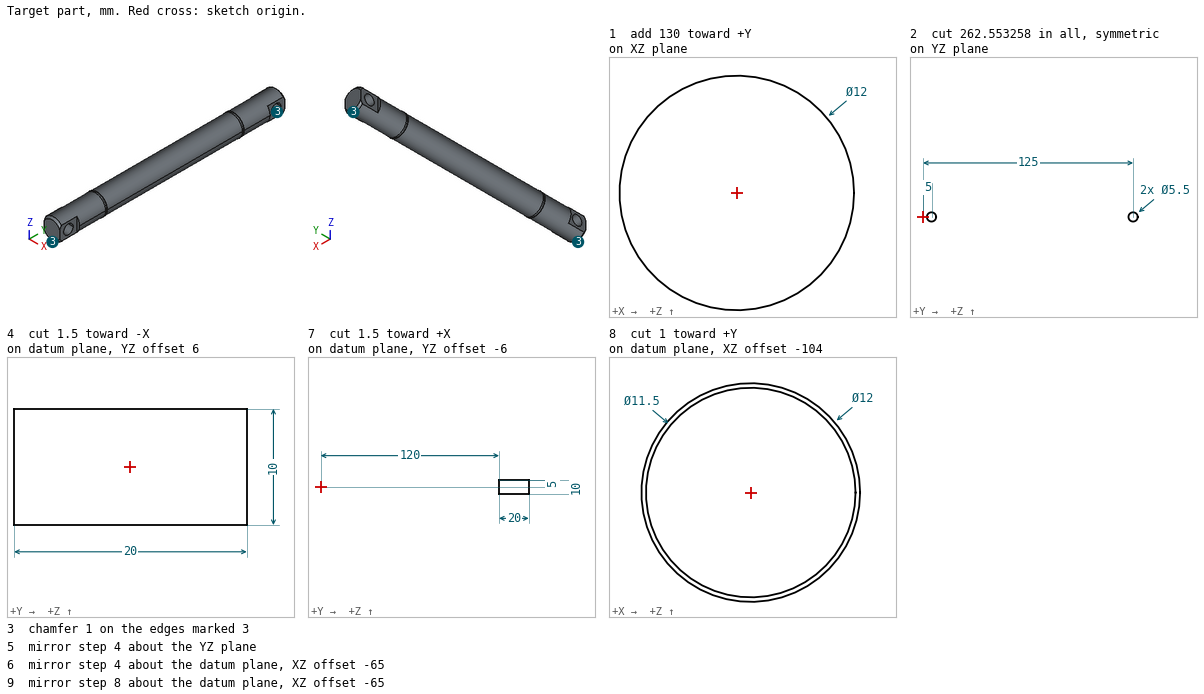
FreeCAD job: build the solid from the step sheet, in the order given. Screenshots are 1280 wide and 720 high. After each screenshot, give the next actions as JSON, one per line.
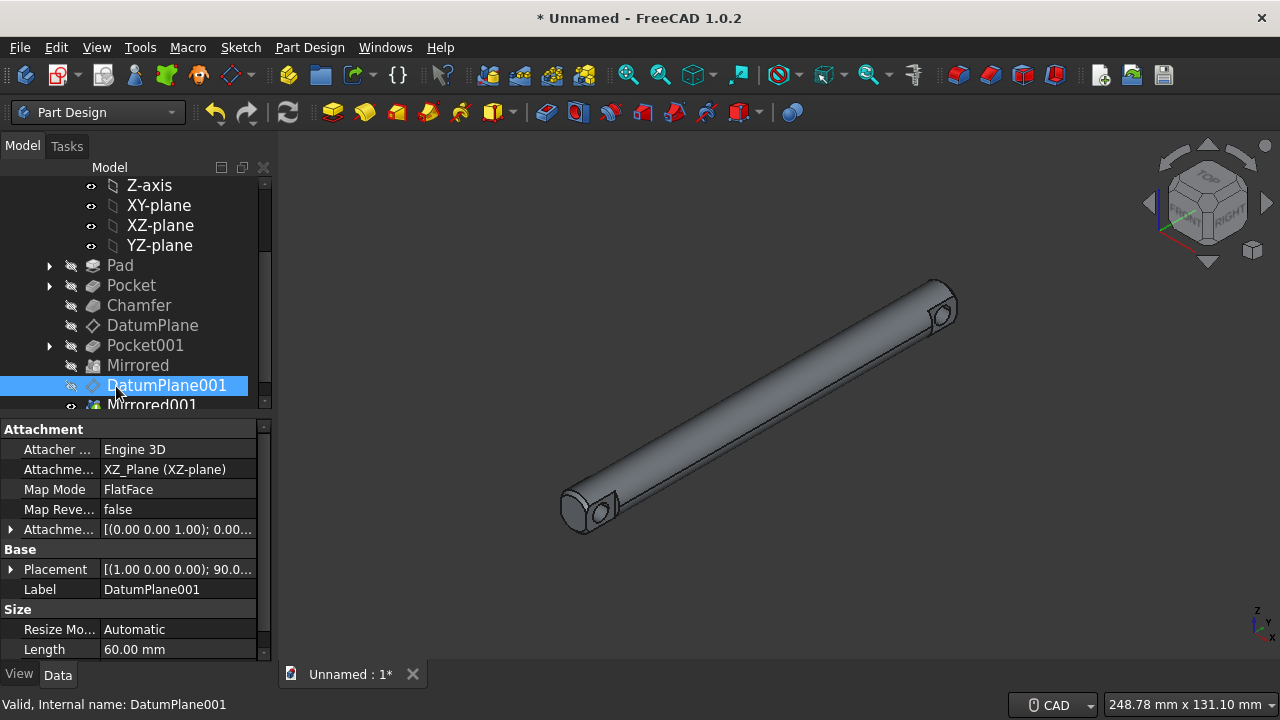
{"action": "scroll", "coordinate": [160, 301], "scroll_direction": "down", "scroll_amount": 3}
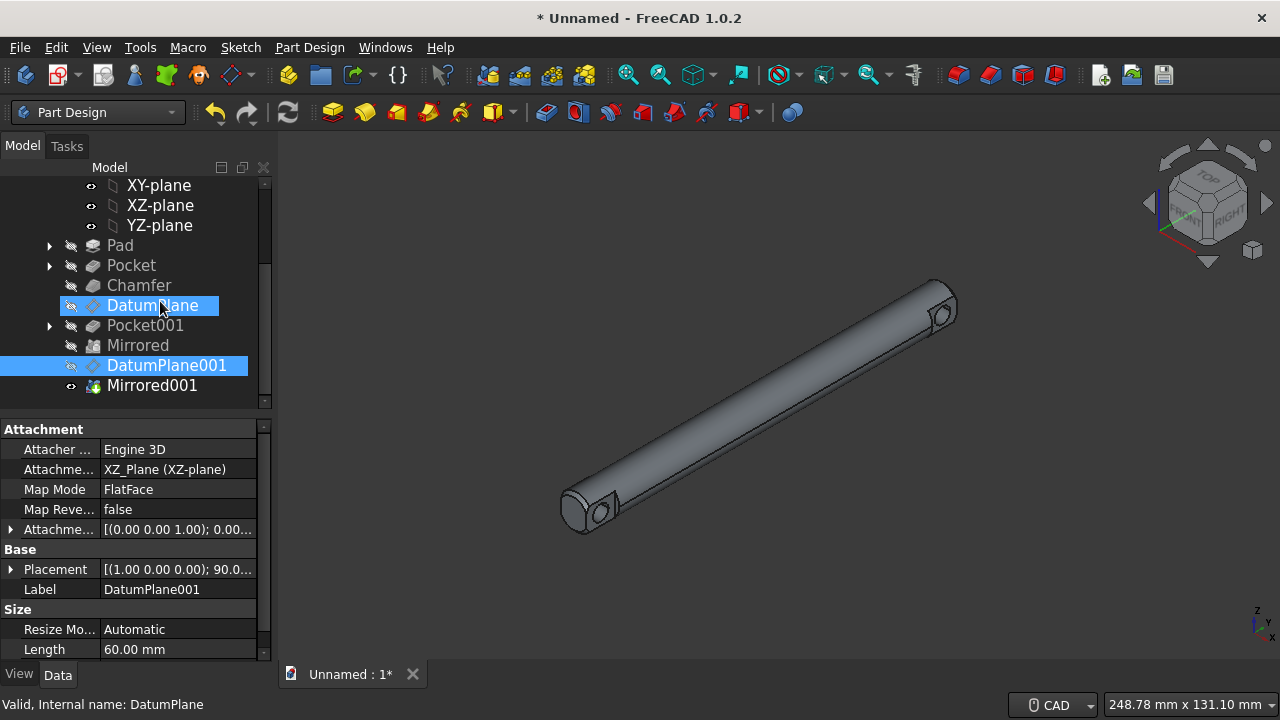
{"action": "scroll", "coordinate": [160, 281], "scroll_direction": "up", "scroll_amount": 15}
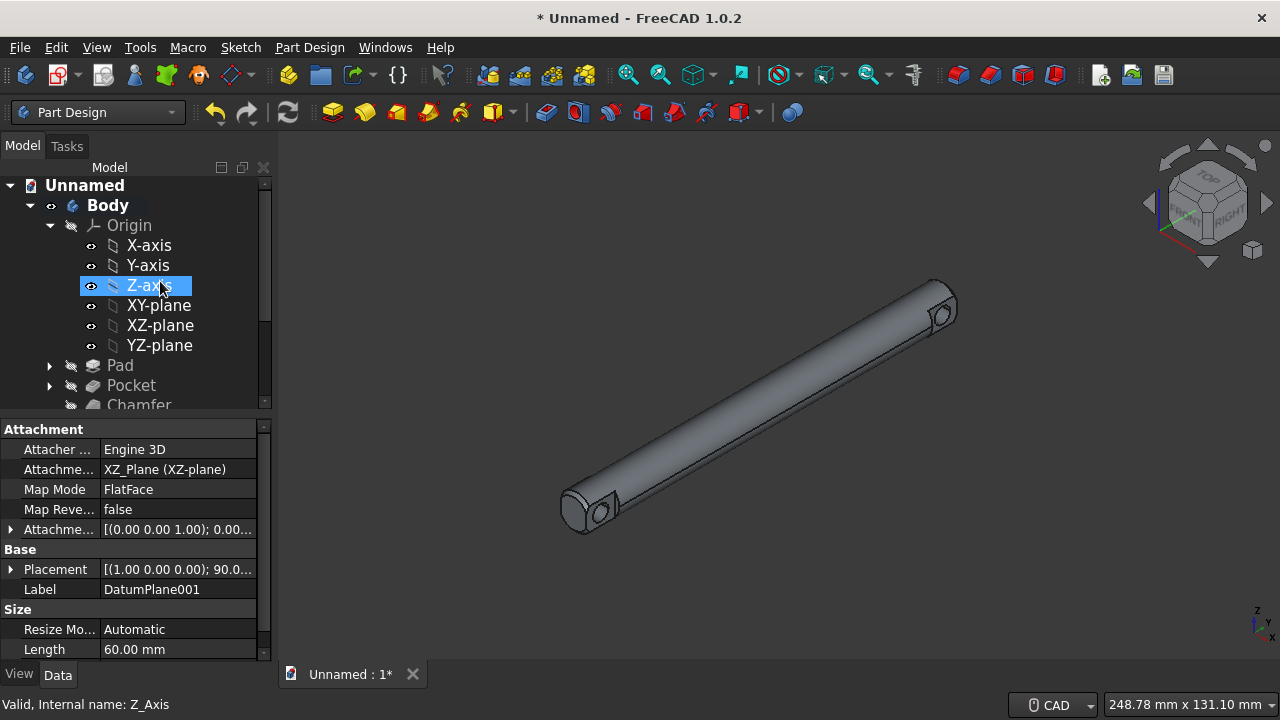
{"action": "left_click", "coordinate": [136, 346]}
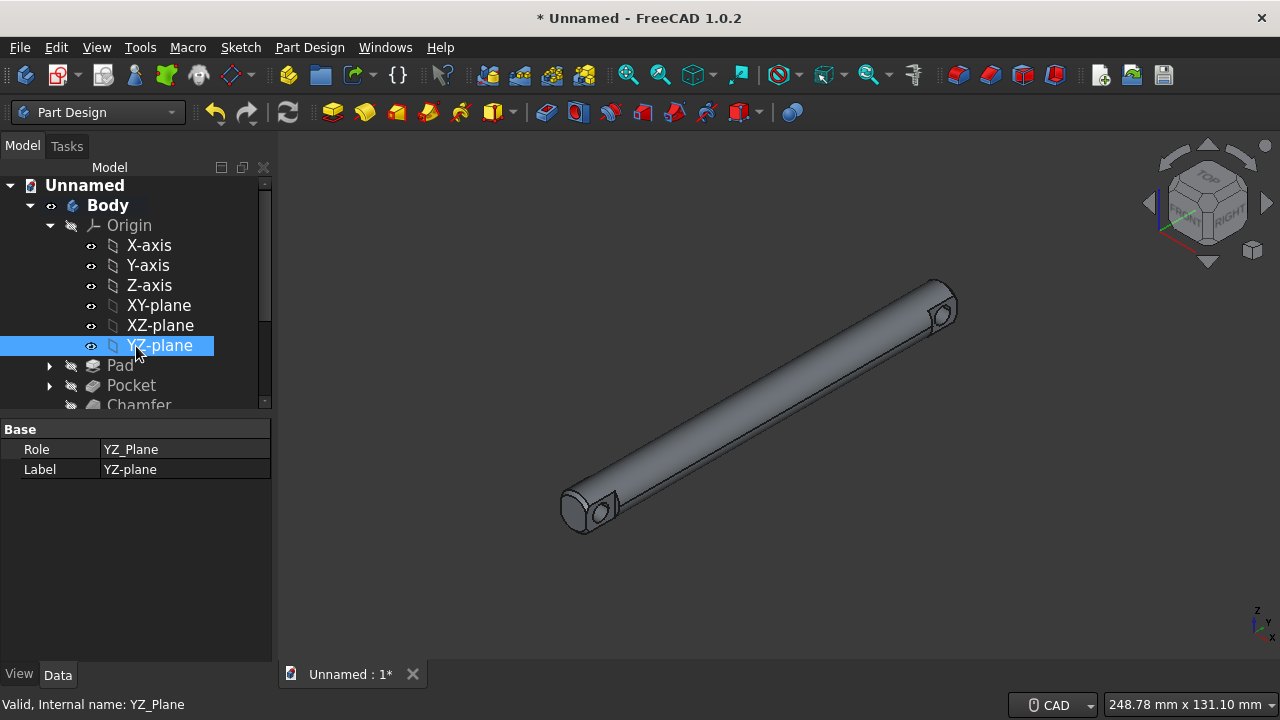
{"action": "left_click", "coordinate": [232, 76]}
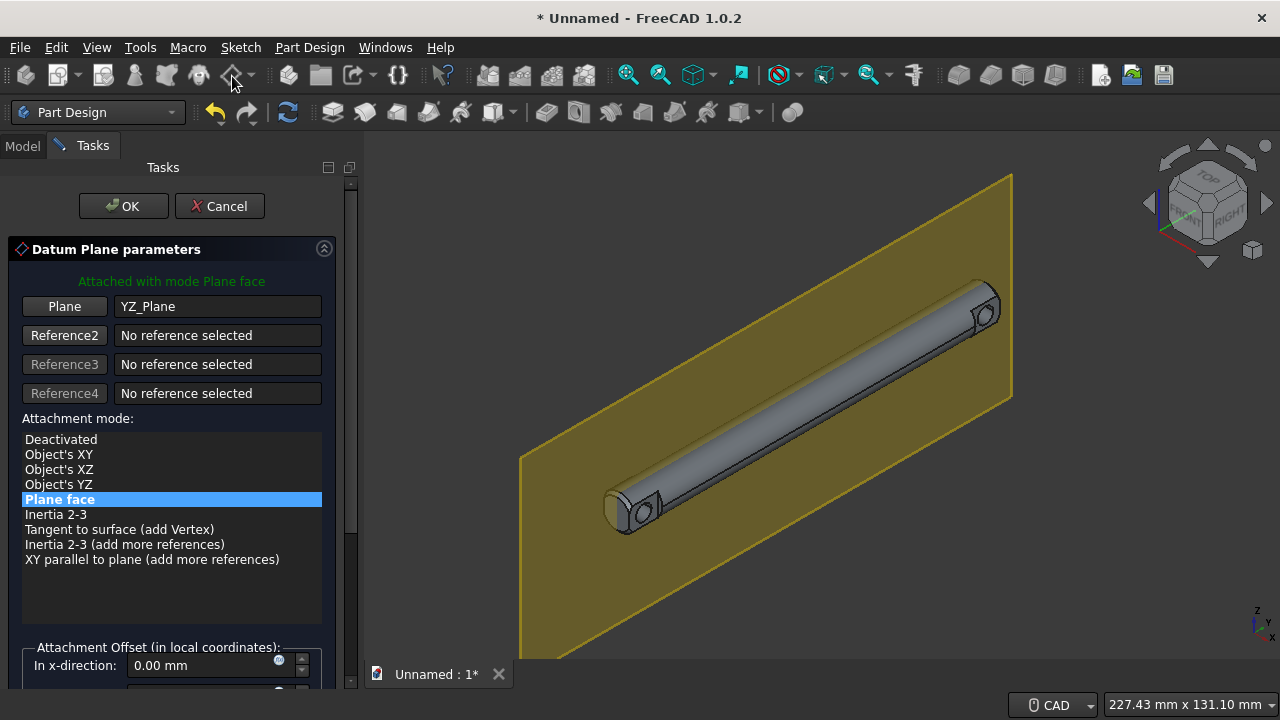
{"action": "scroll", "coordinate": [351, 432], "scroll_direction": "down", "scroll_amount": 2}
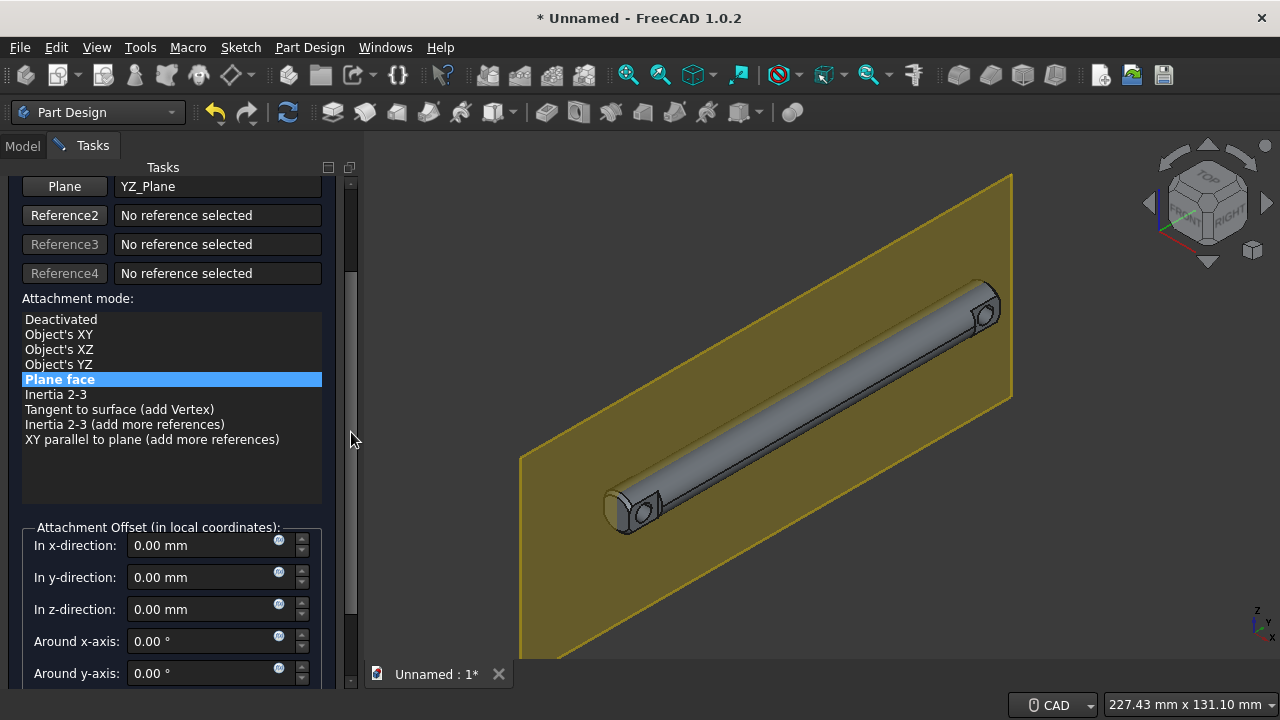
{"action": "triple_click", "coordinate": [210, 609]}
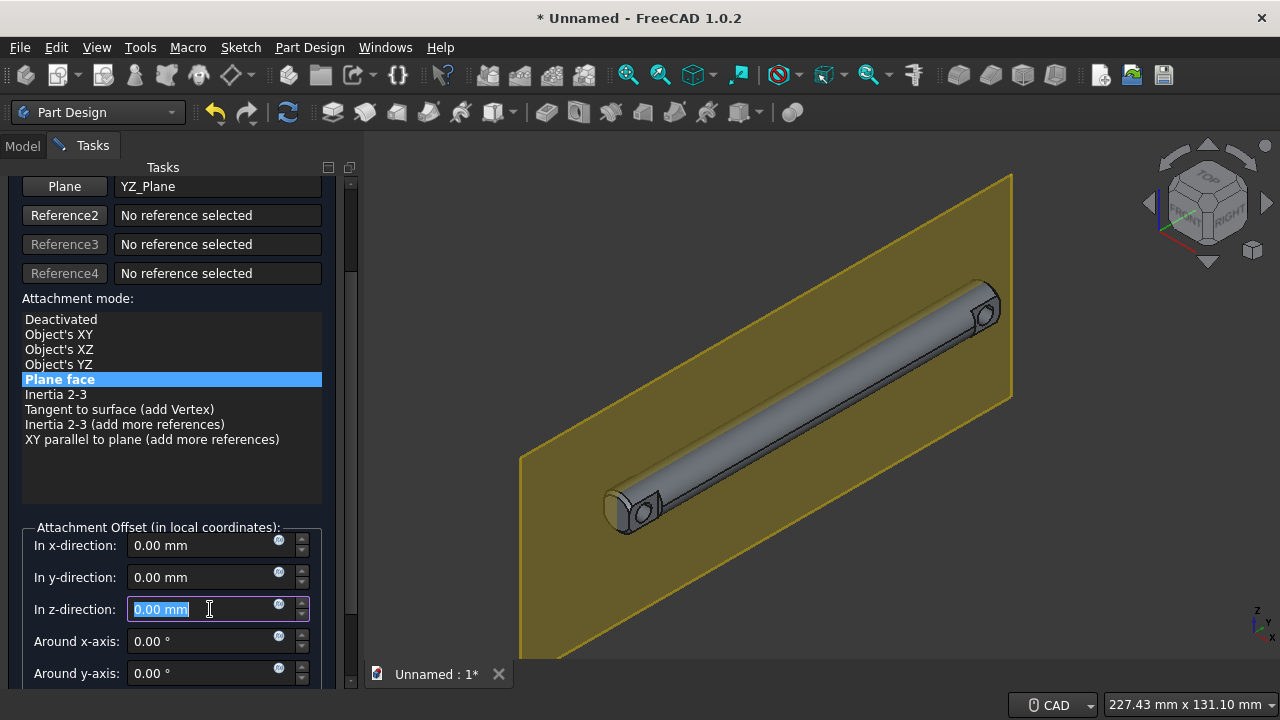
{"action": "type", "text": "-6"}
{"action": "key", "text": "Tab"}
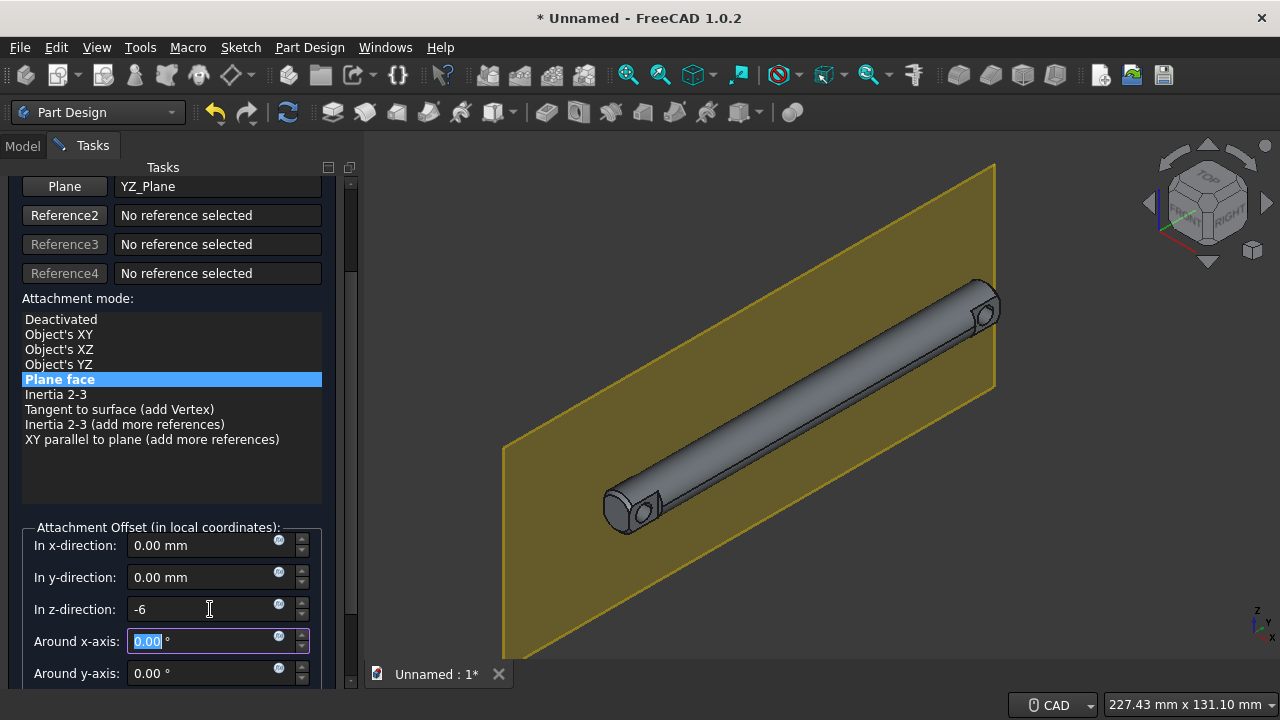
{"action": "scroll", "coordinate": [351, 432], "scroll_direction": "up", "scroll_amount": 3}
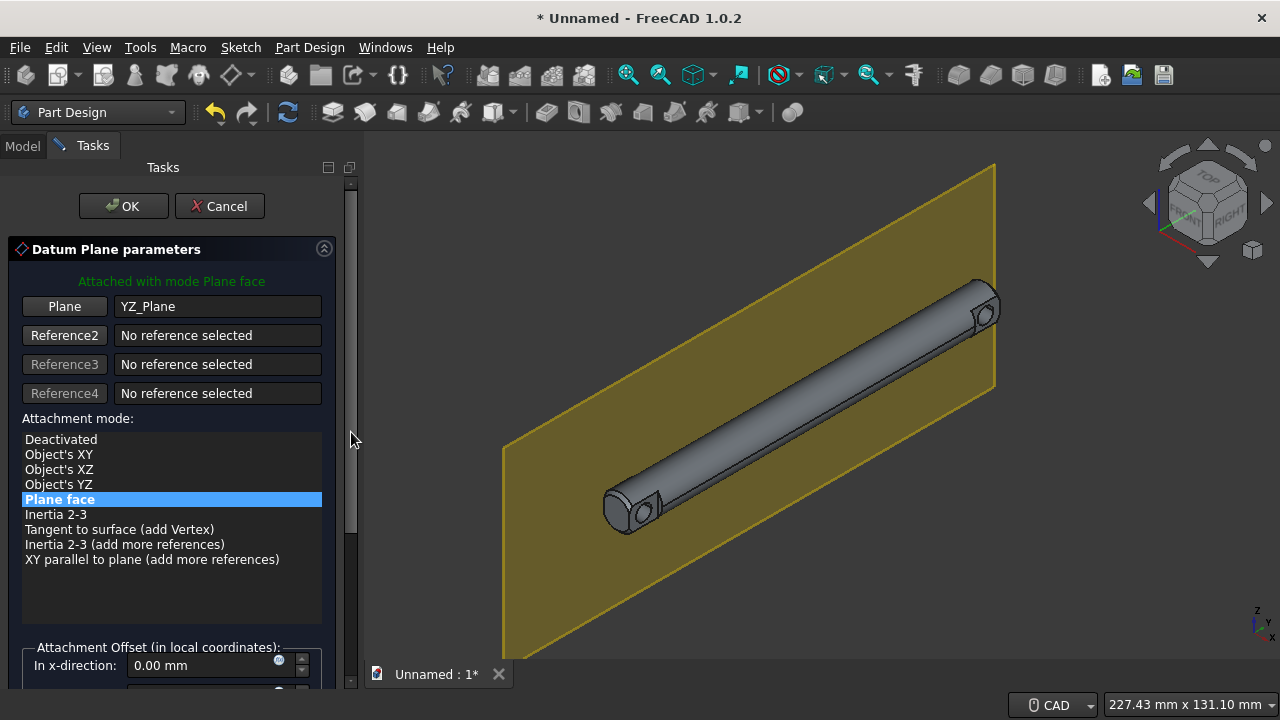
{"action": "left_click", "coordinate": [124, 206]}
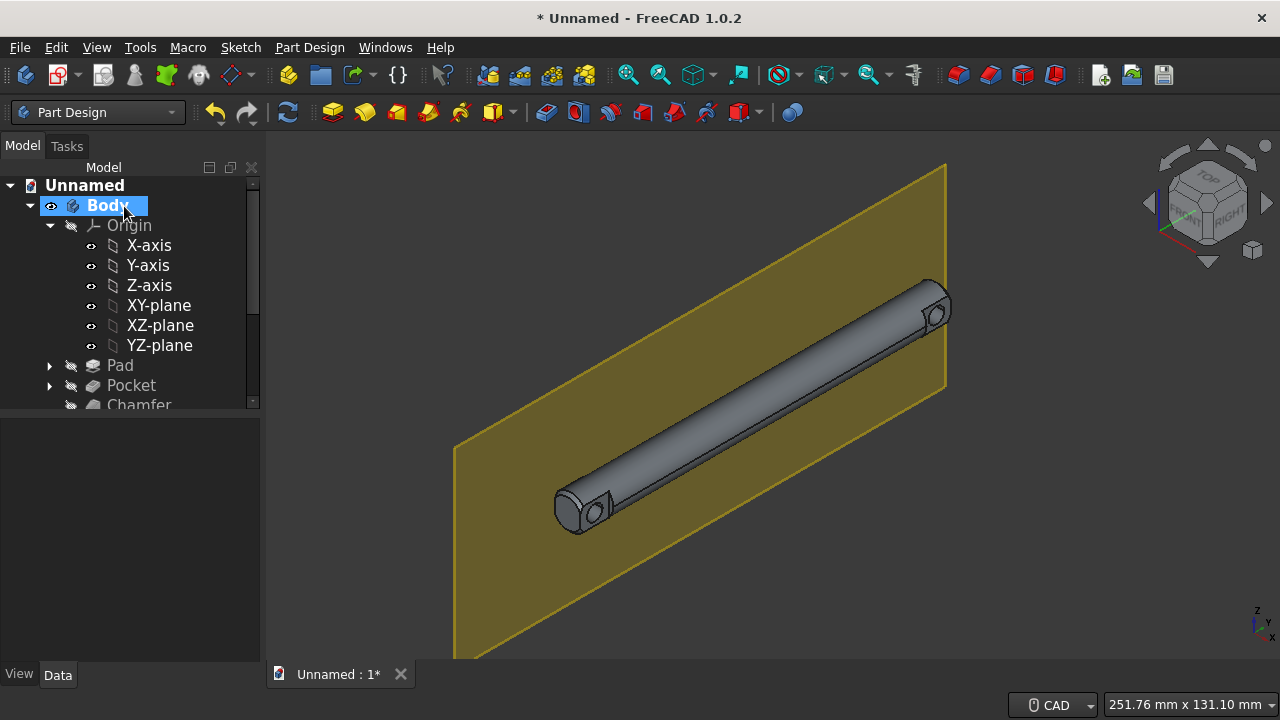
{"action": "scroll", "coordinate": [100, 301], "scroll_direction": "down", "scroll_amount": 3}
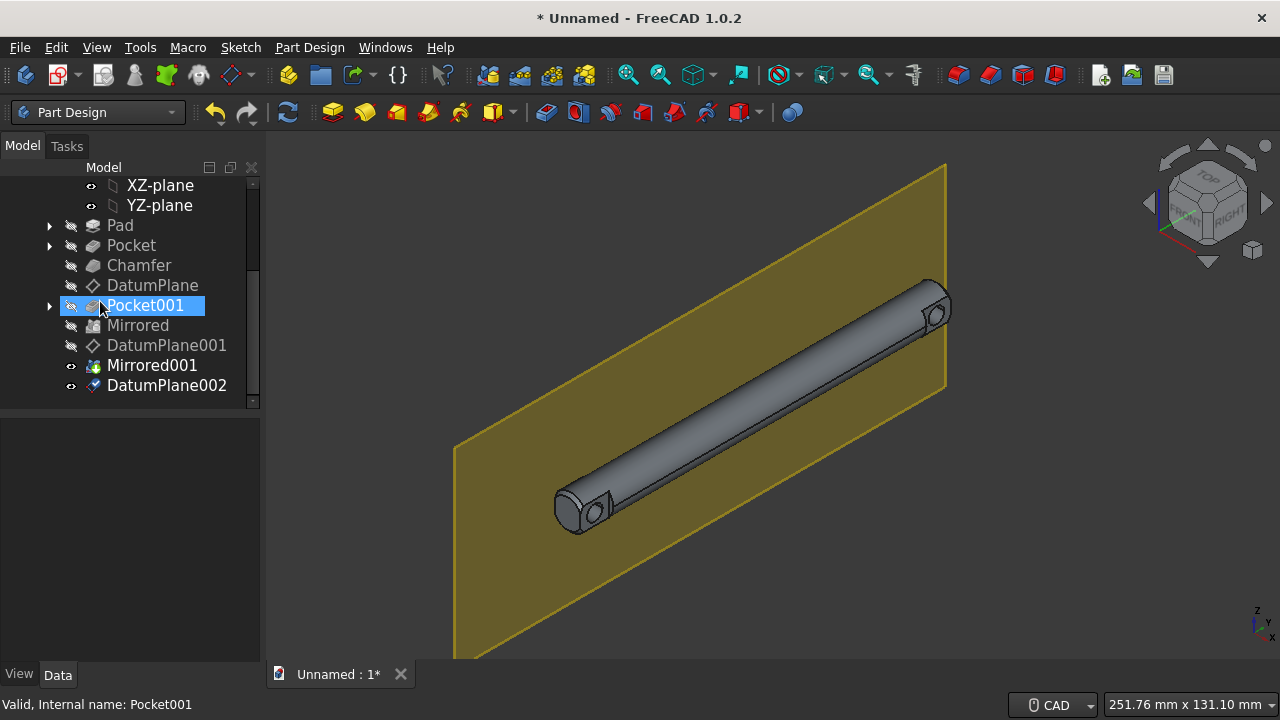
{"action": "left_click", "coordinate": [116, 386]}